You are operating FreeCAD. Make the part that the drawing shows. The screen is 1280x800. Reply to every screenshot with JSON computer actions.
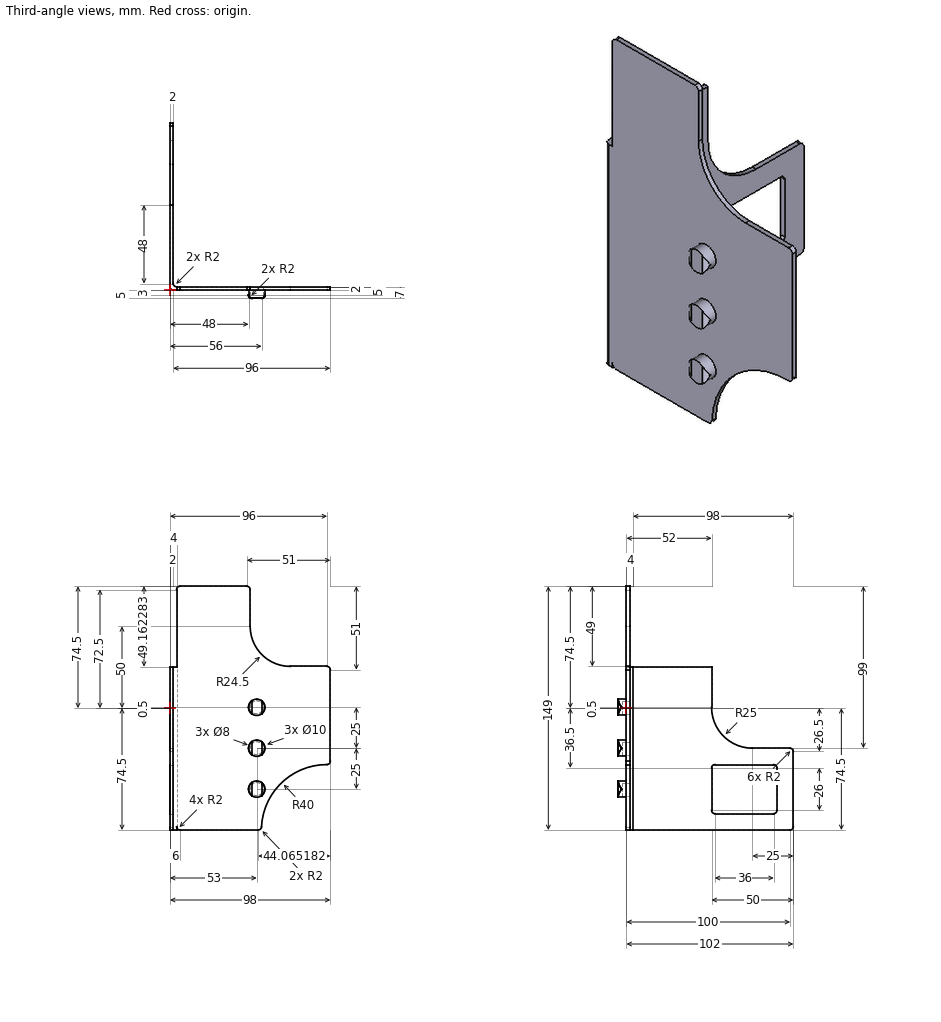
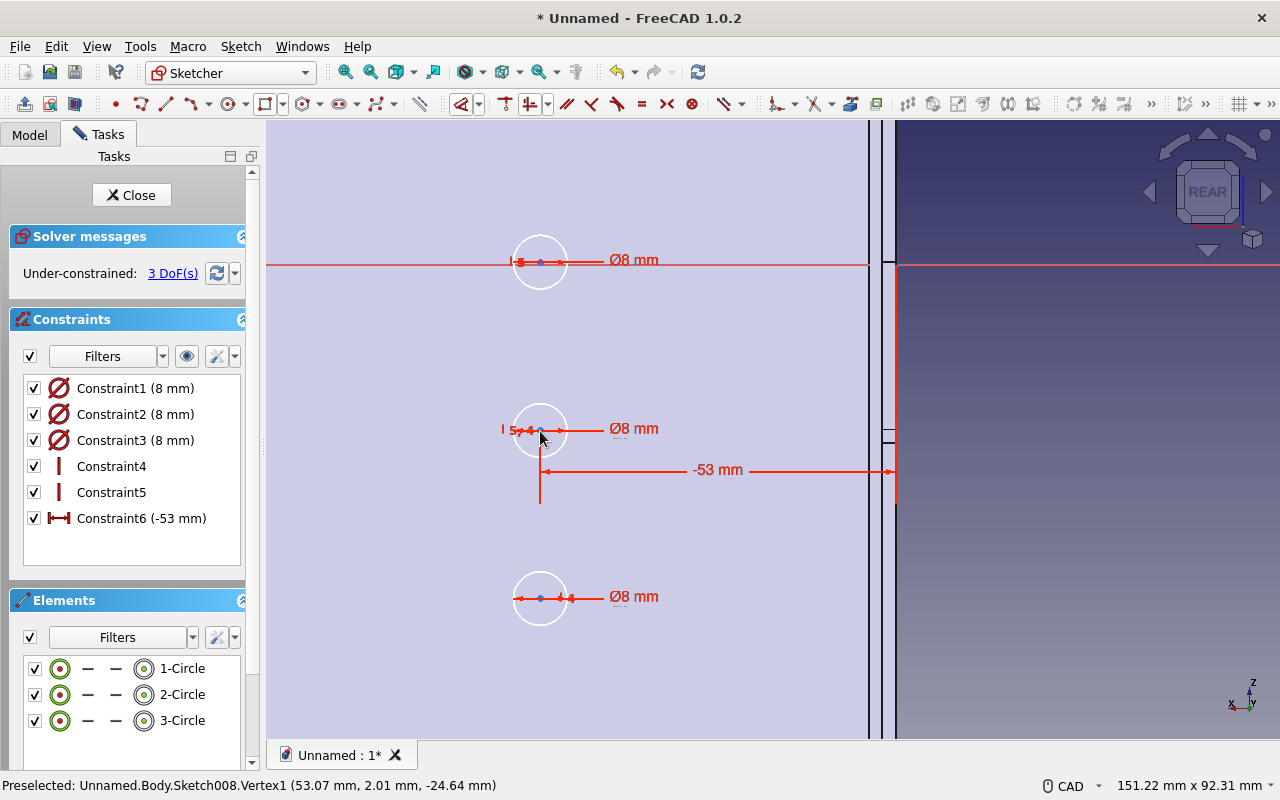
{"action": "scroll", "coordinate": [540, 262], "scroll_direction": "up", "scroll_amount": 13}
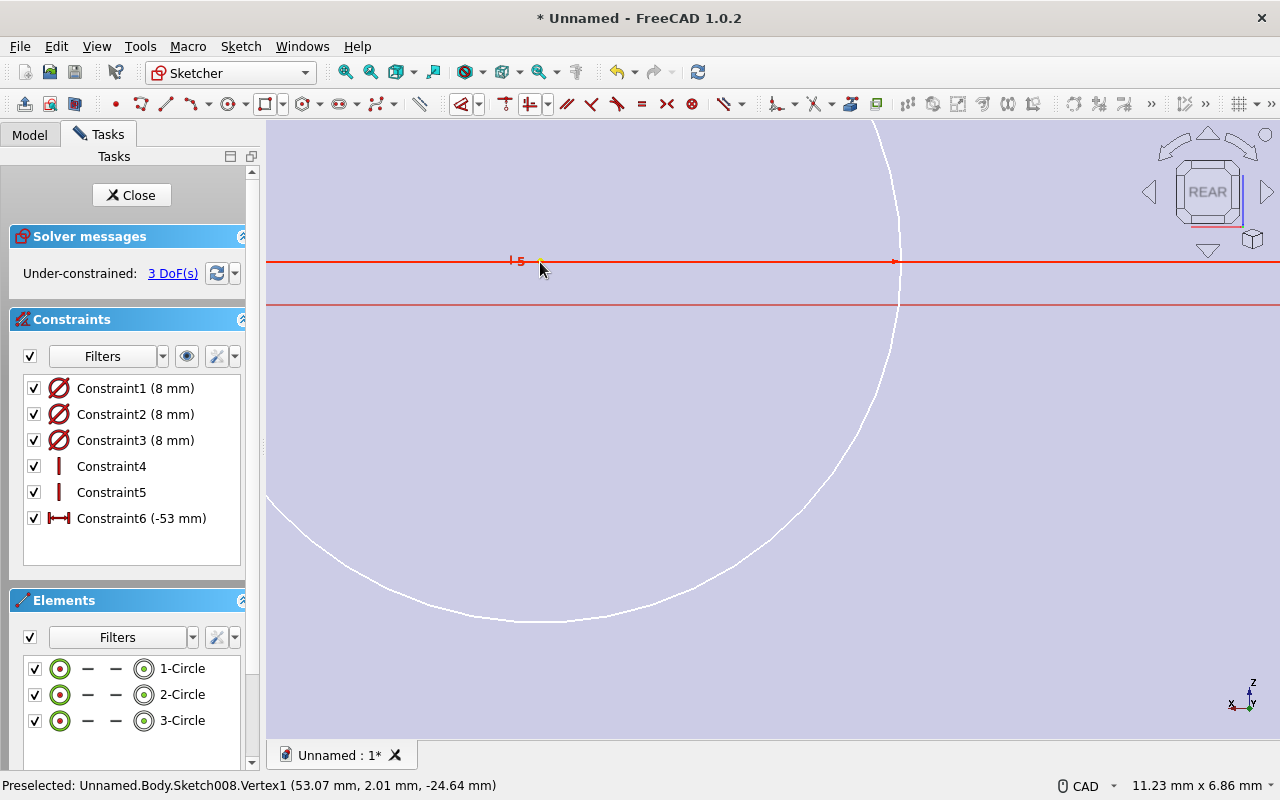
{"action": "left_click", "coordinate": [540, 262]}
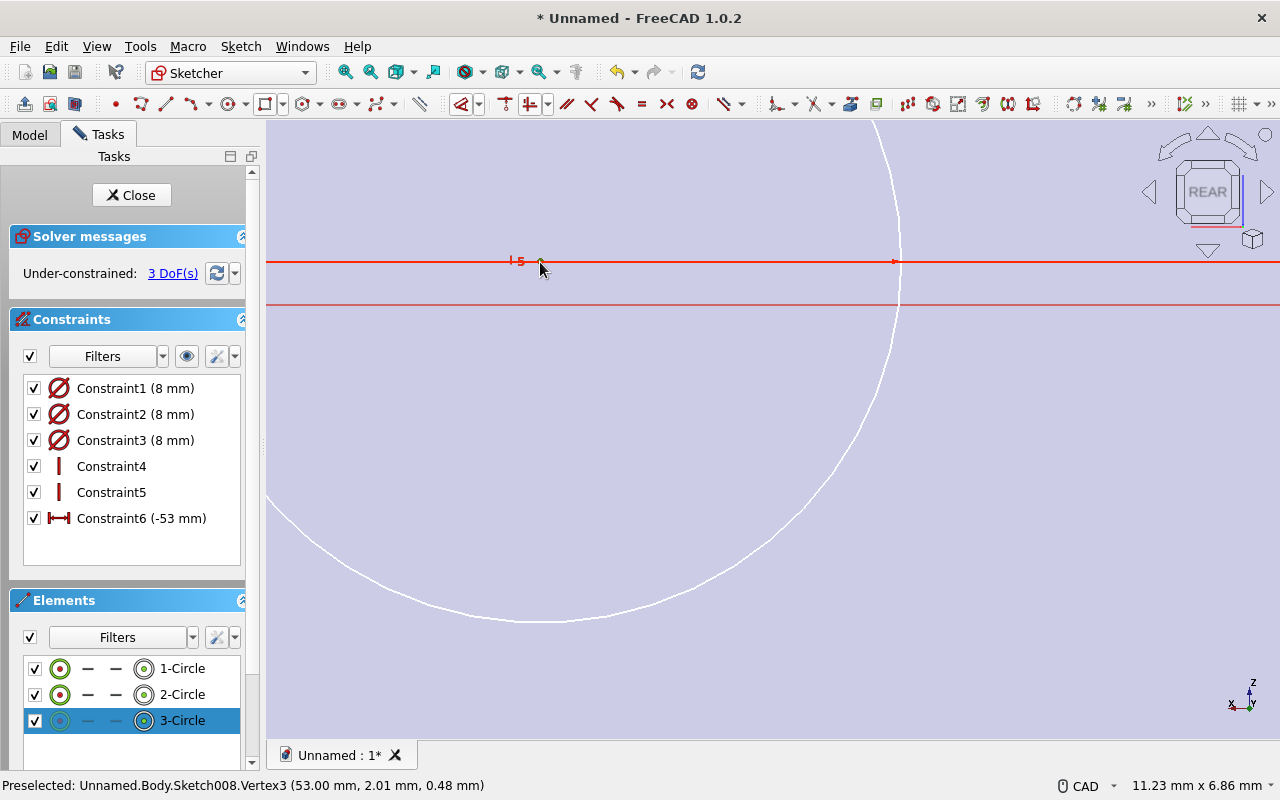
{"action": "key", "text": "i"}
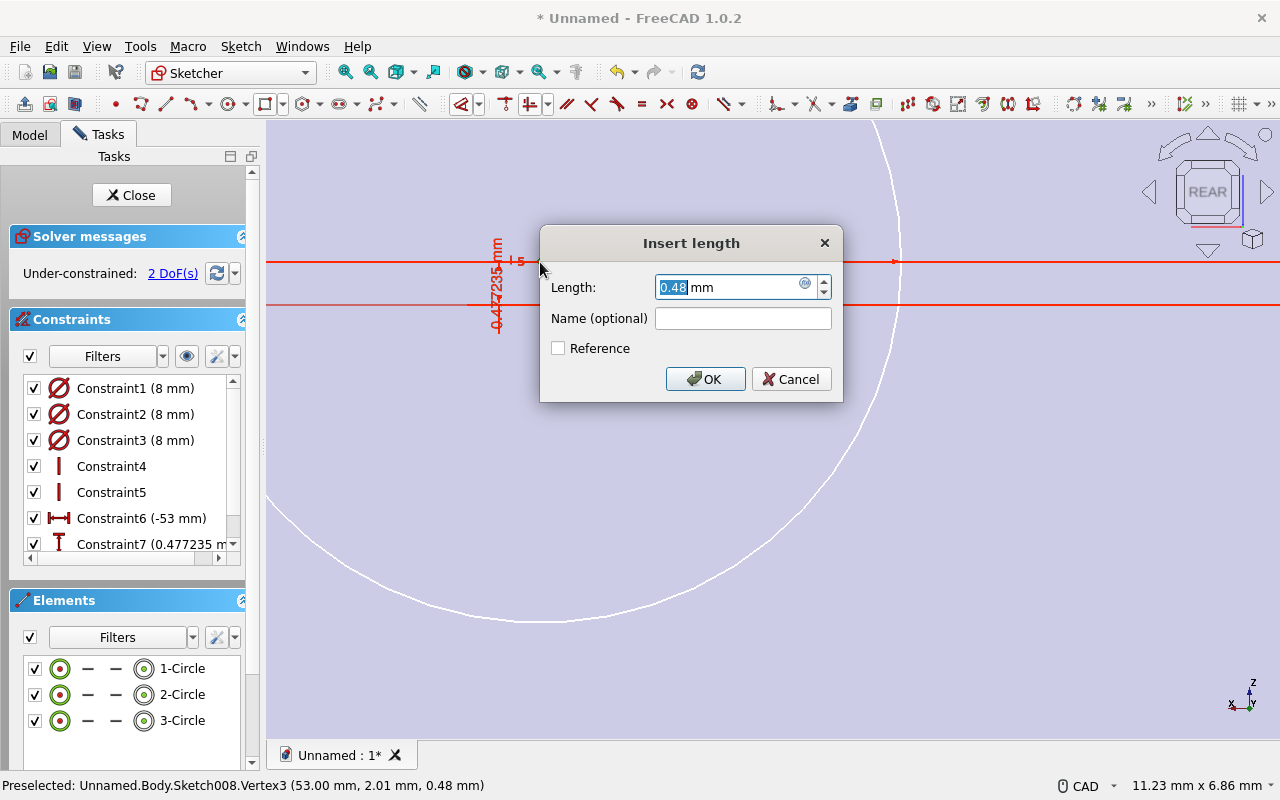
{"action": "type", "text": "0.5"}
{"action": "key", "text": "Return"}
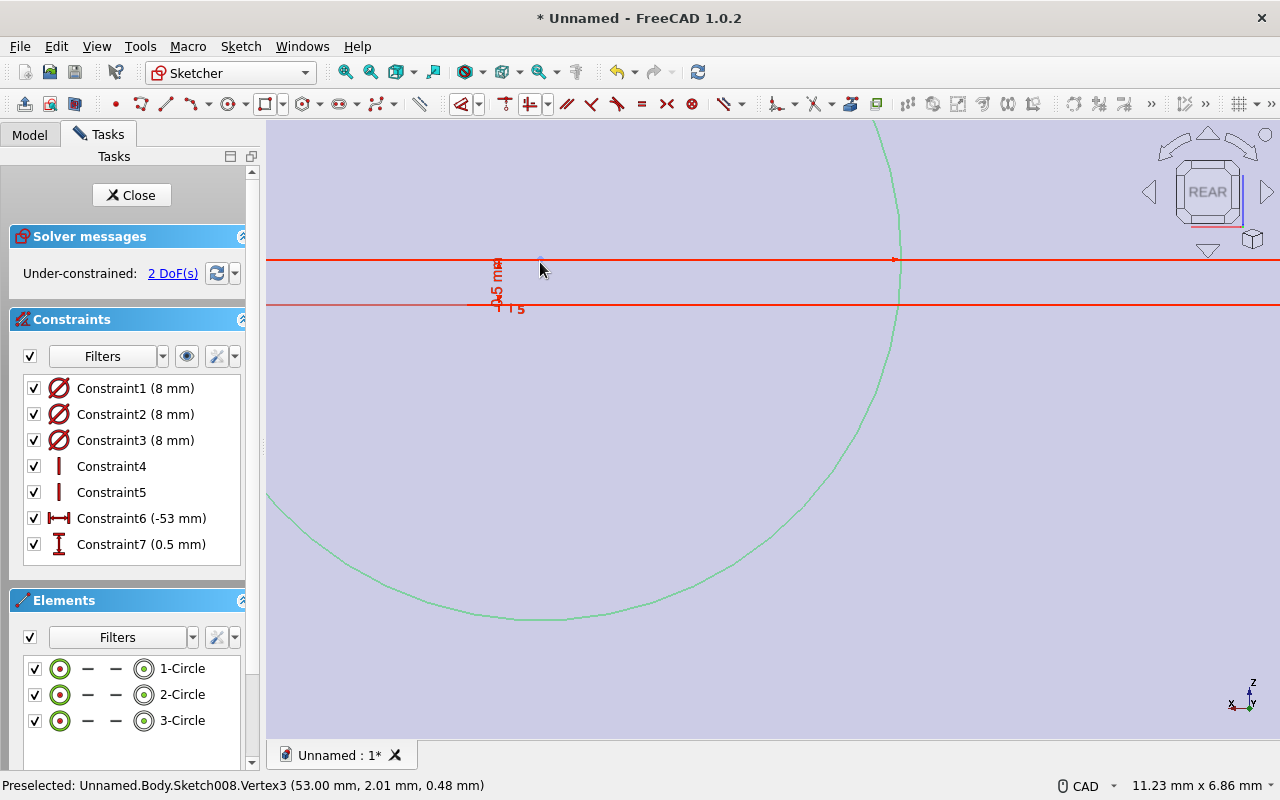
{"action": "scroll", "coordinate": [540, 262], "scroll_direction": "down", "scroll_amount": 13}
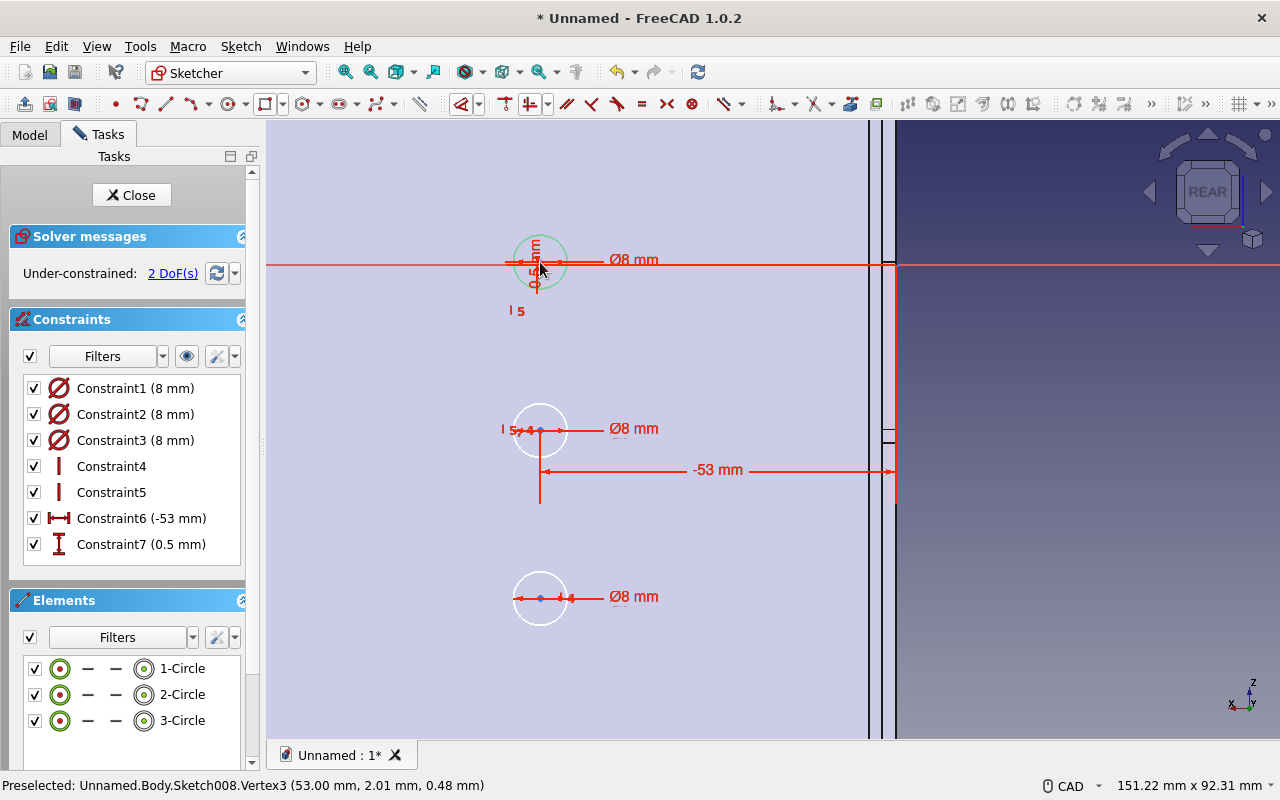
{"action": "left_click", "coordinate": [540, 431]}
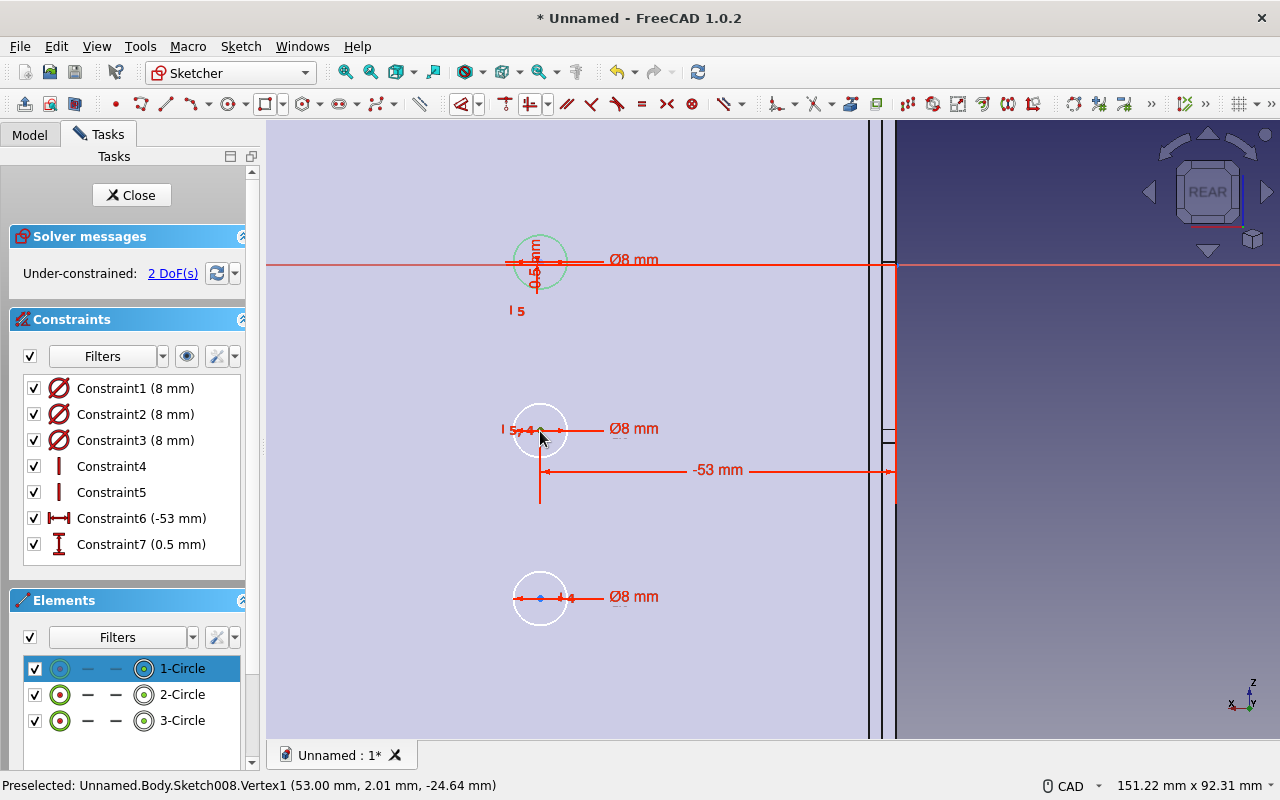
{"action": "left_click", "coordinate": [540, 599]}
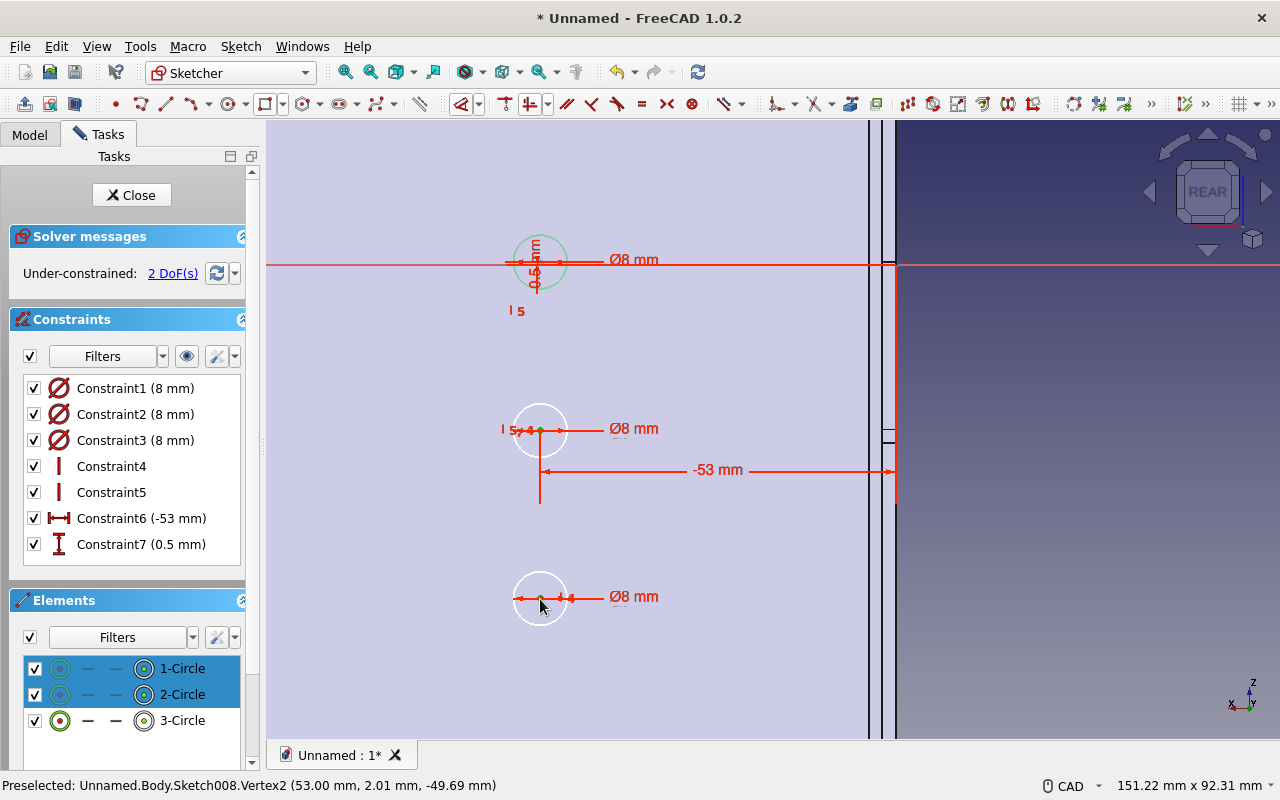
{"action": "left_click", "coordinate": [478, 104]}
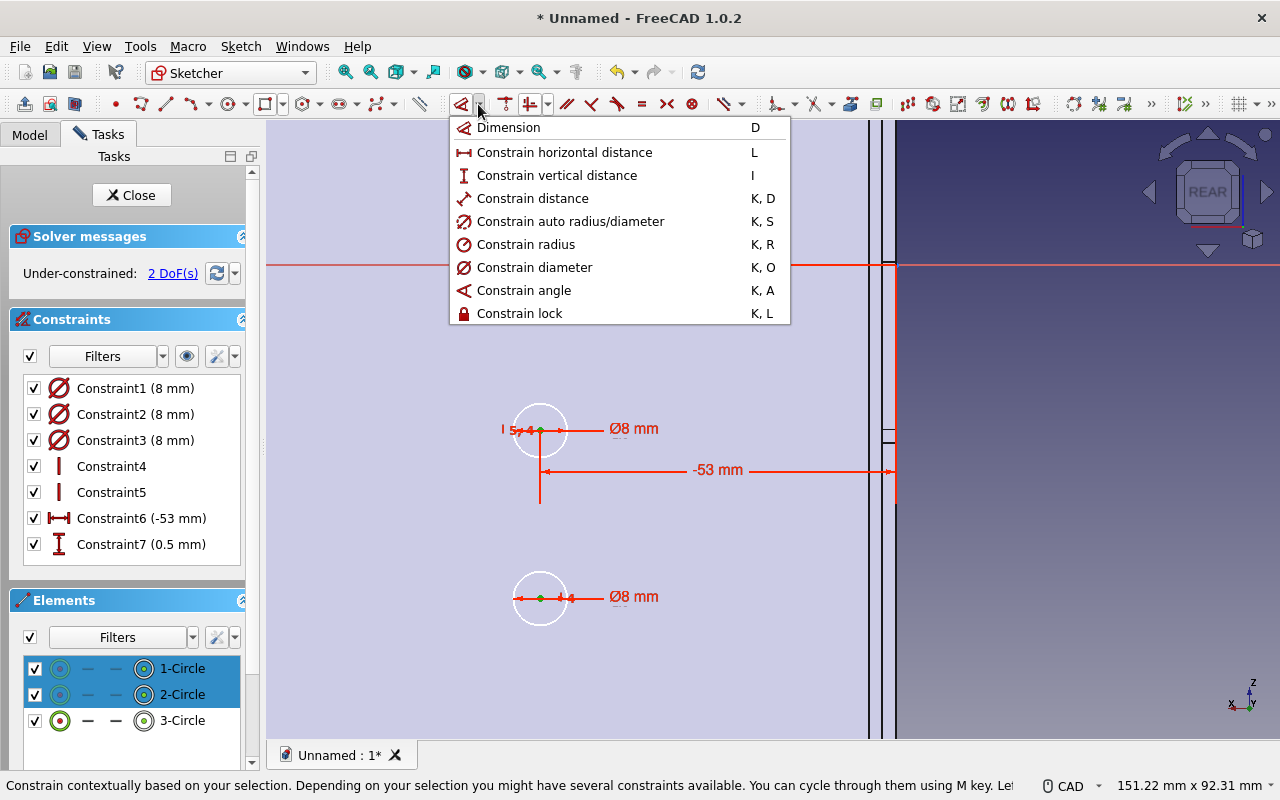
{"action": "left_click", "coordinate": [620, 176]}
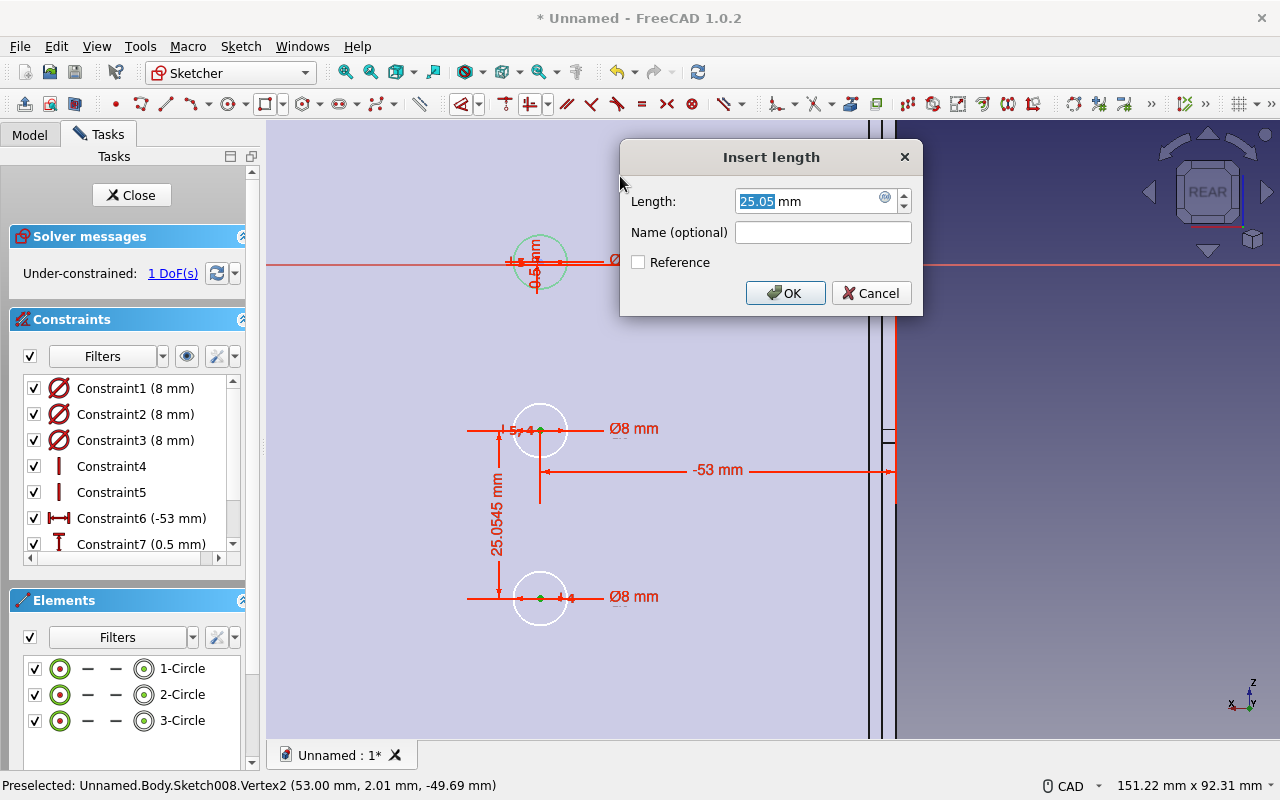
{"action": "type", "text": "25"}
{"action": "key", "text": "Return"}